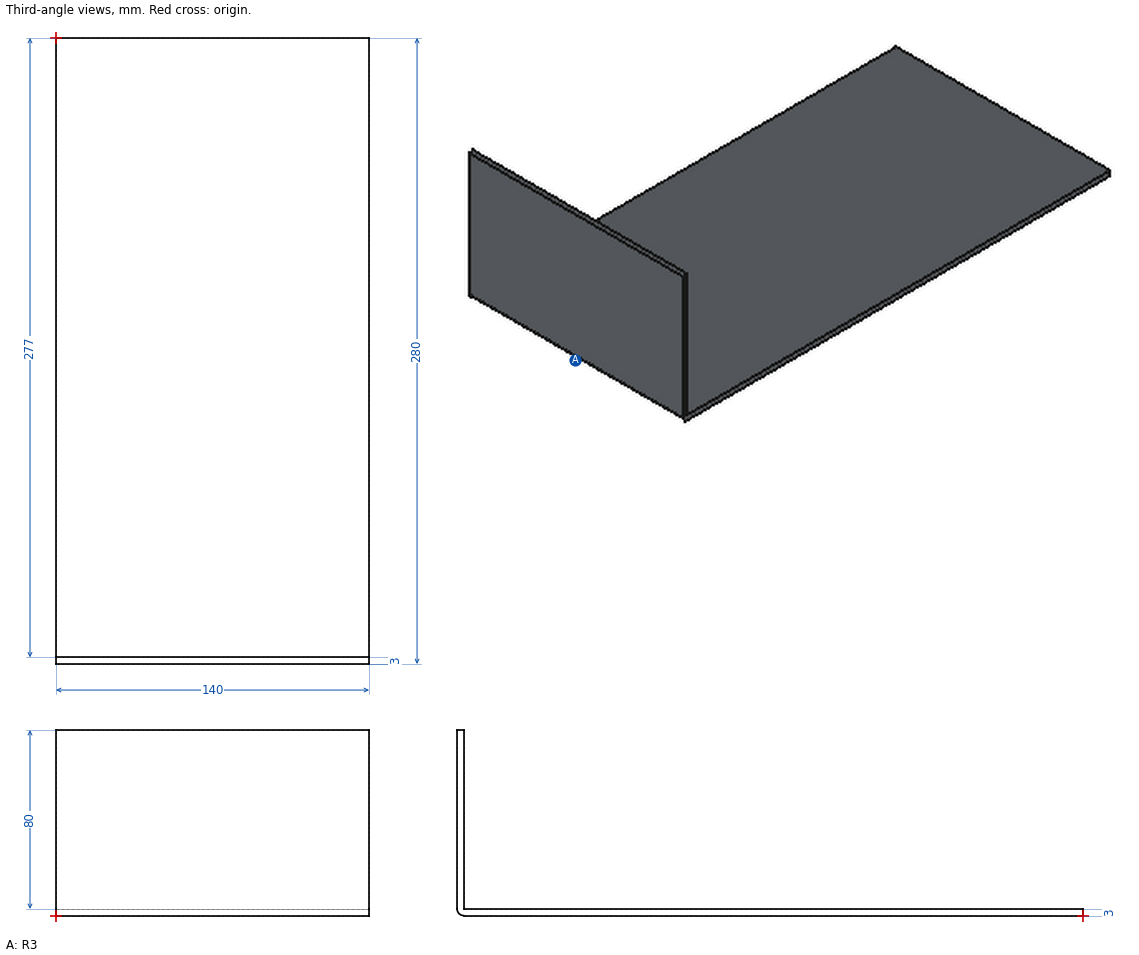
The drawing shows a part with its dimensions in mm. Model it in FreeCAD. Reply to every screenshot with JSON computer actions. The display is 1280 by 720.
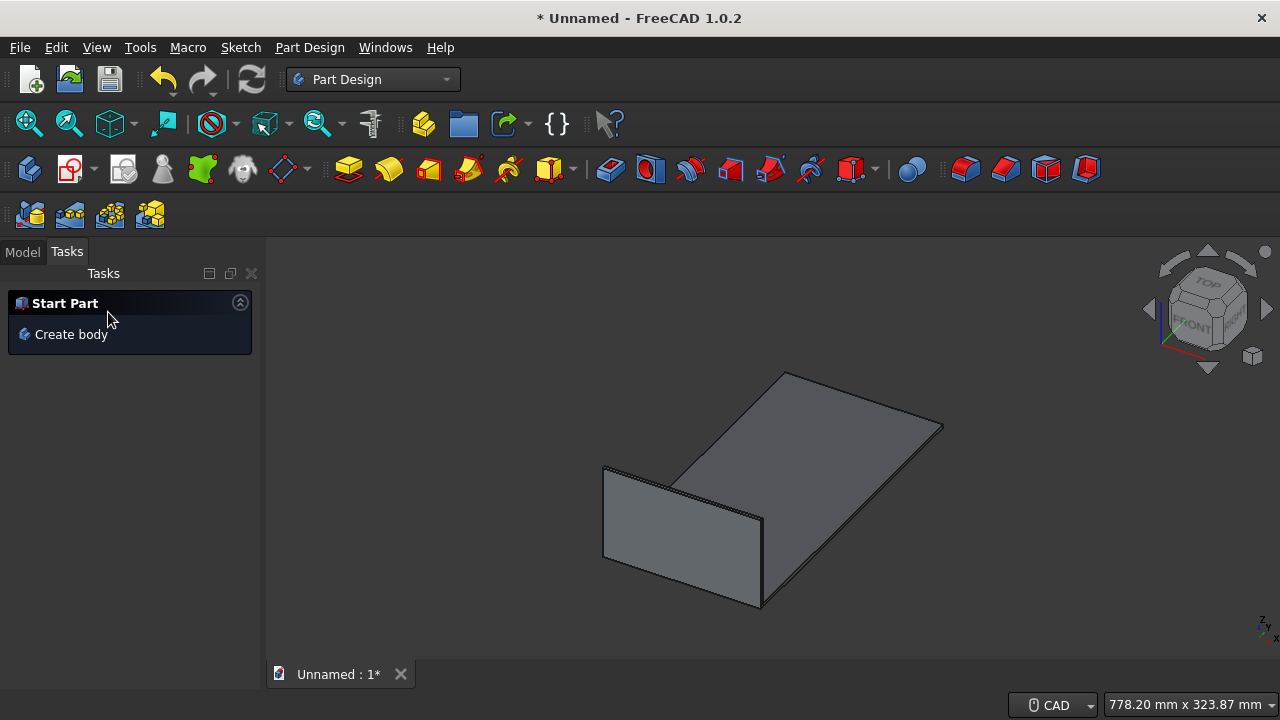
{"action": "key", "text": "0"}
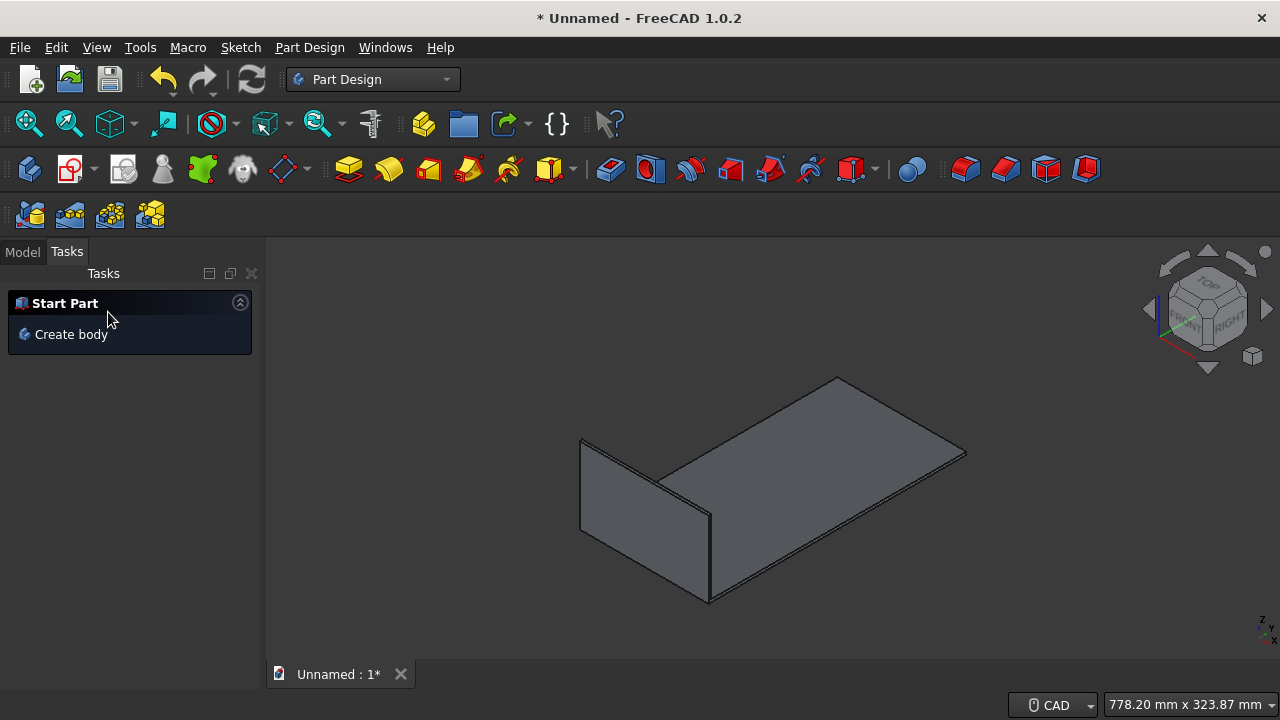
{"action": "key", "text": "2"}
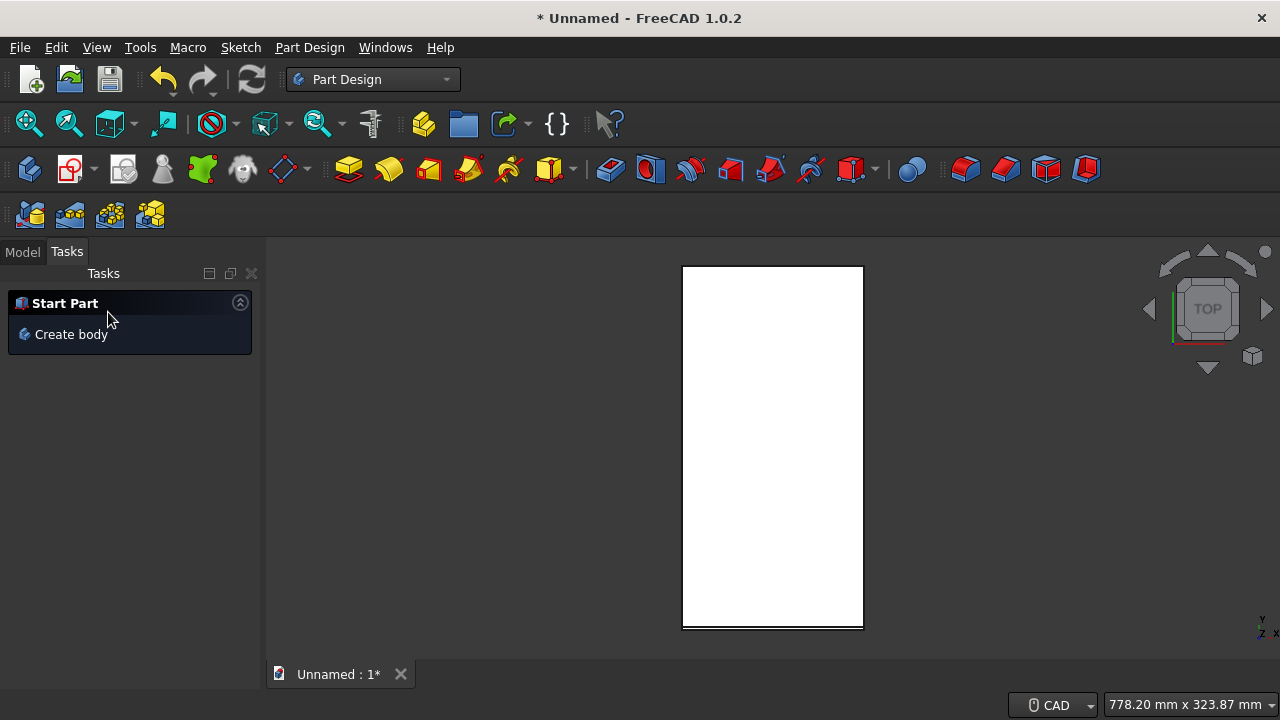
{"action": "key", "text": "1"}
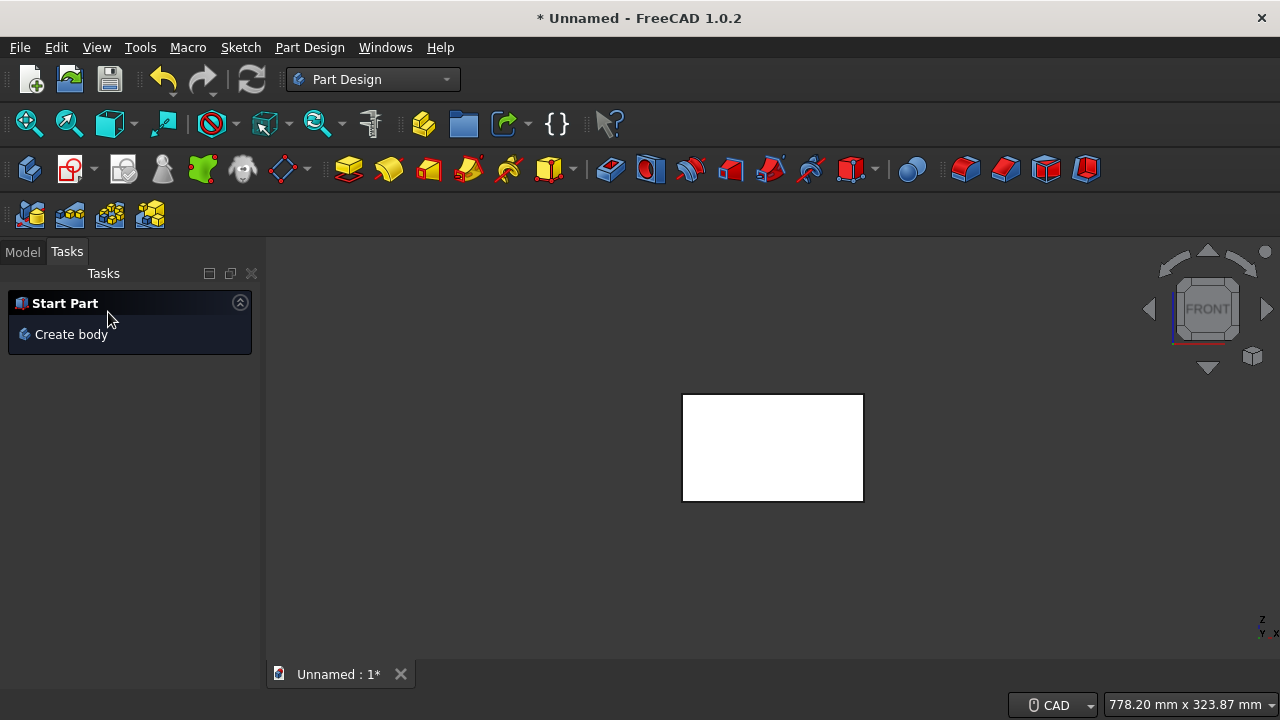
{"action": "key", "text": "v f"}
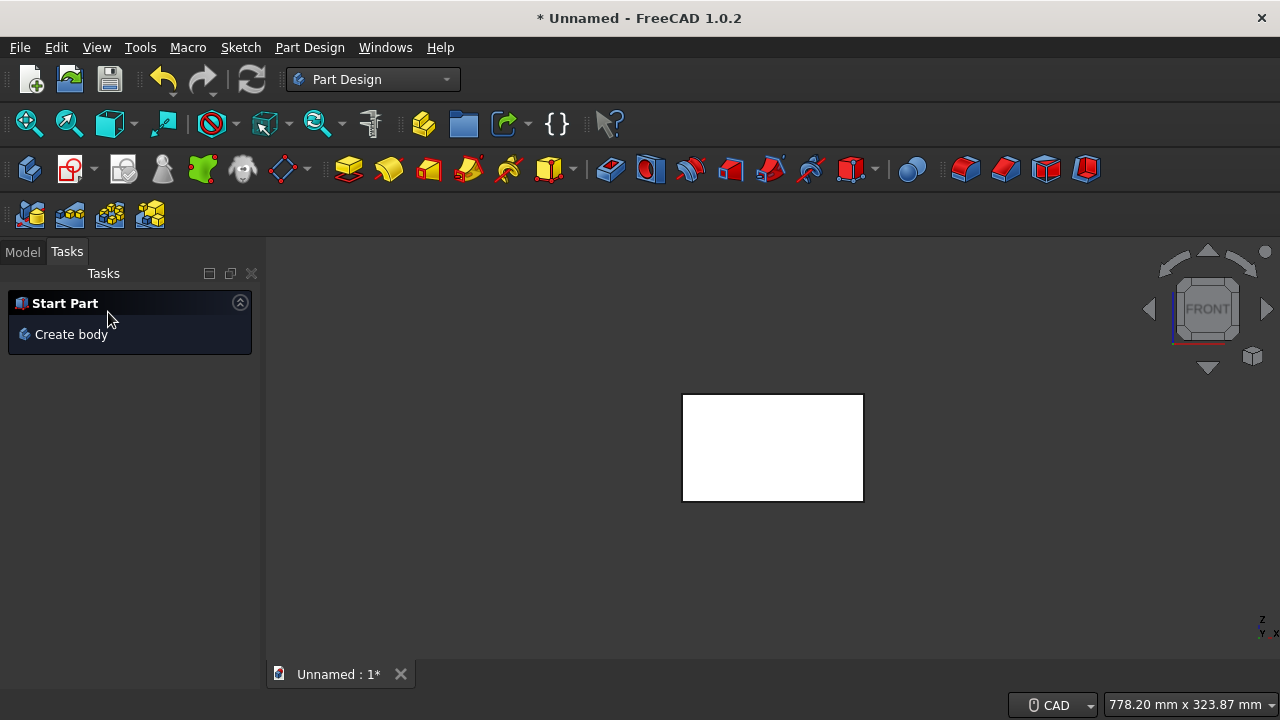
{"action": "left_click", "coordinate": [773, 501]}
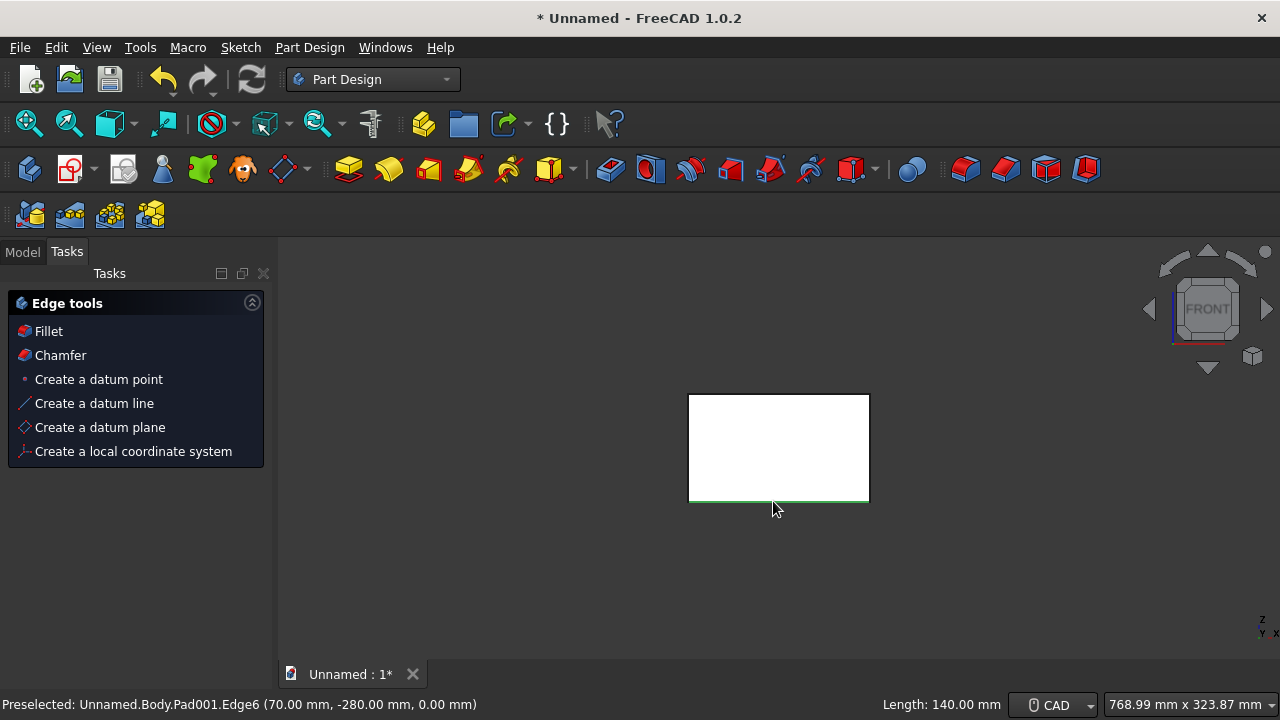
{"action": "left_click", "coordinate": [966, 170]}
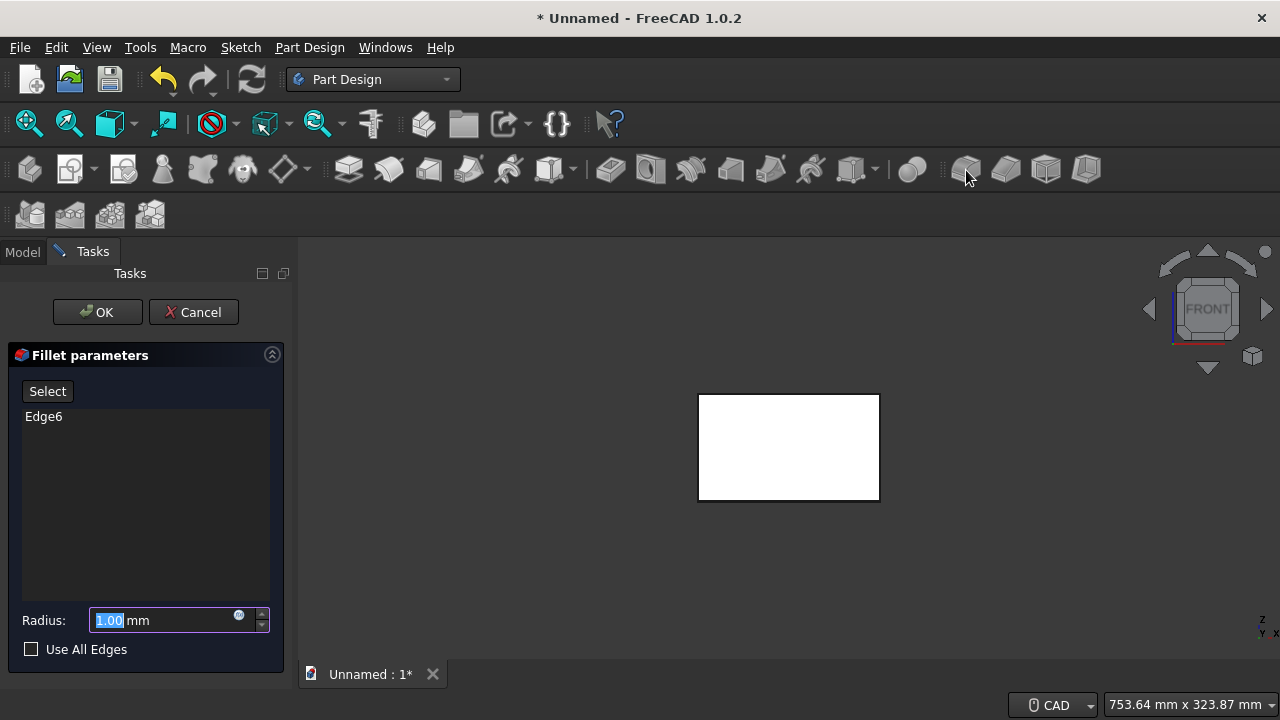
{"action": "type", "text": "3"}
{"action": "key", "text": "Tab"}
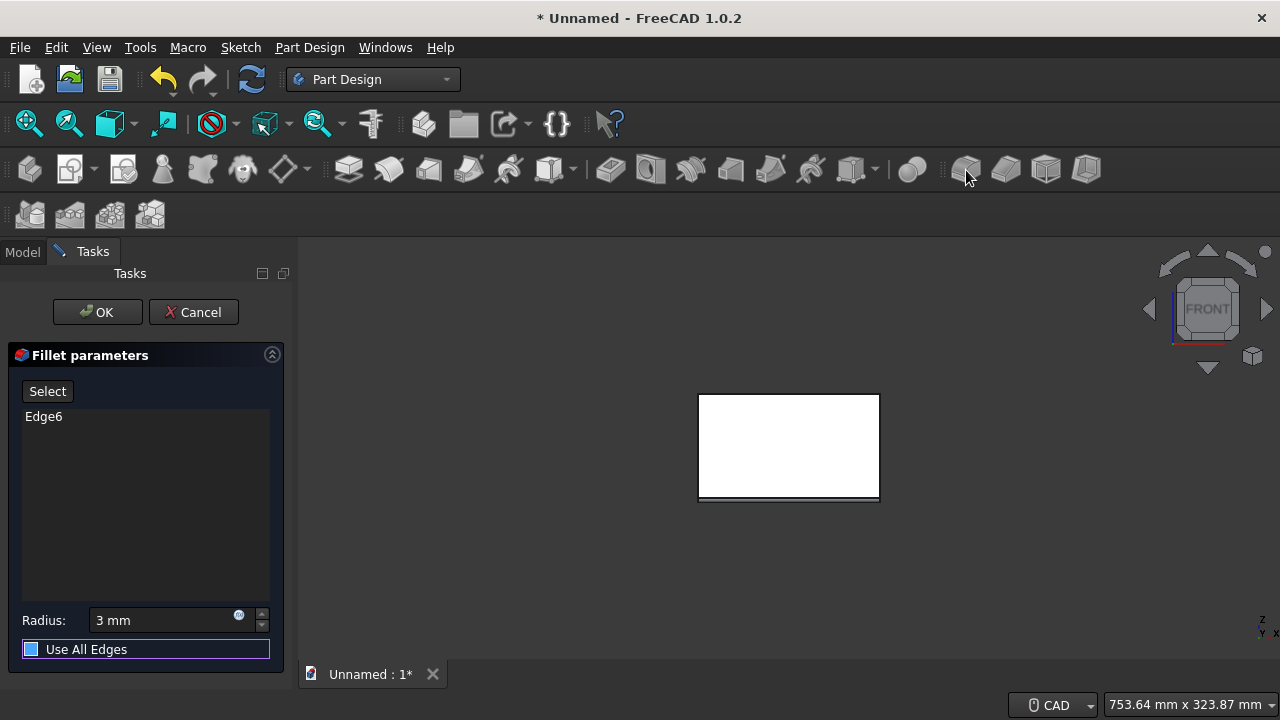
{"action": "left_click", "coordinate": [98, 312]}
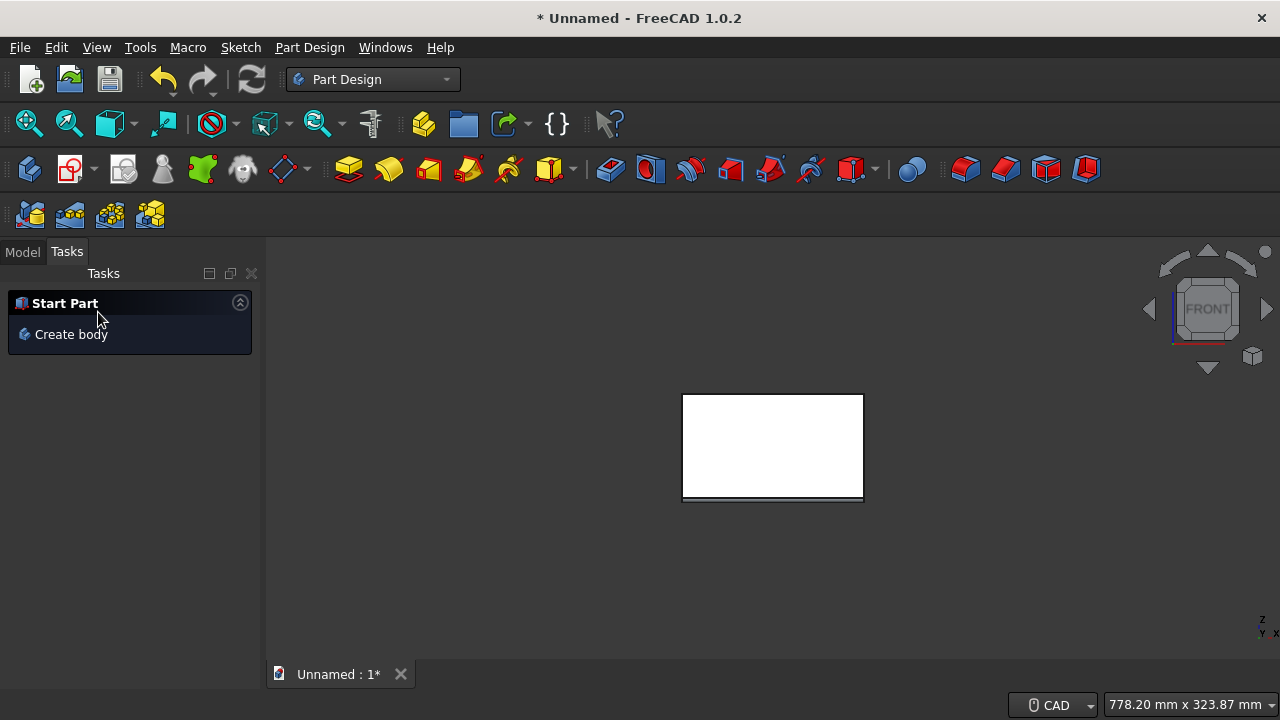
{"action": "key", "text": "0"}